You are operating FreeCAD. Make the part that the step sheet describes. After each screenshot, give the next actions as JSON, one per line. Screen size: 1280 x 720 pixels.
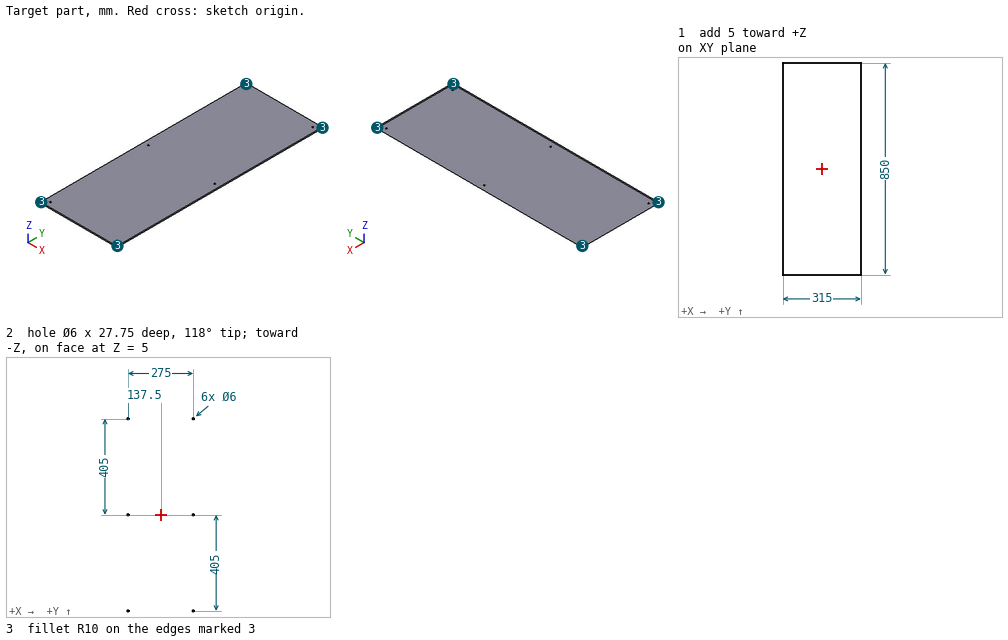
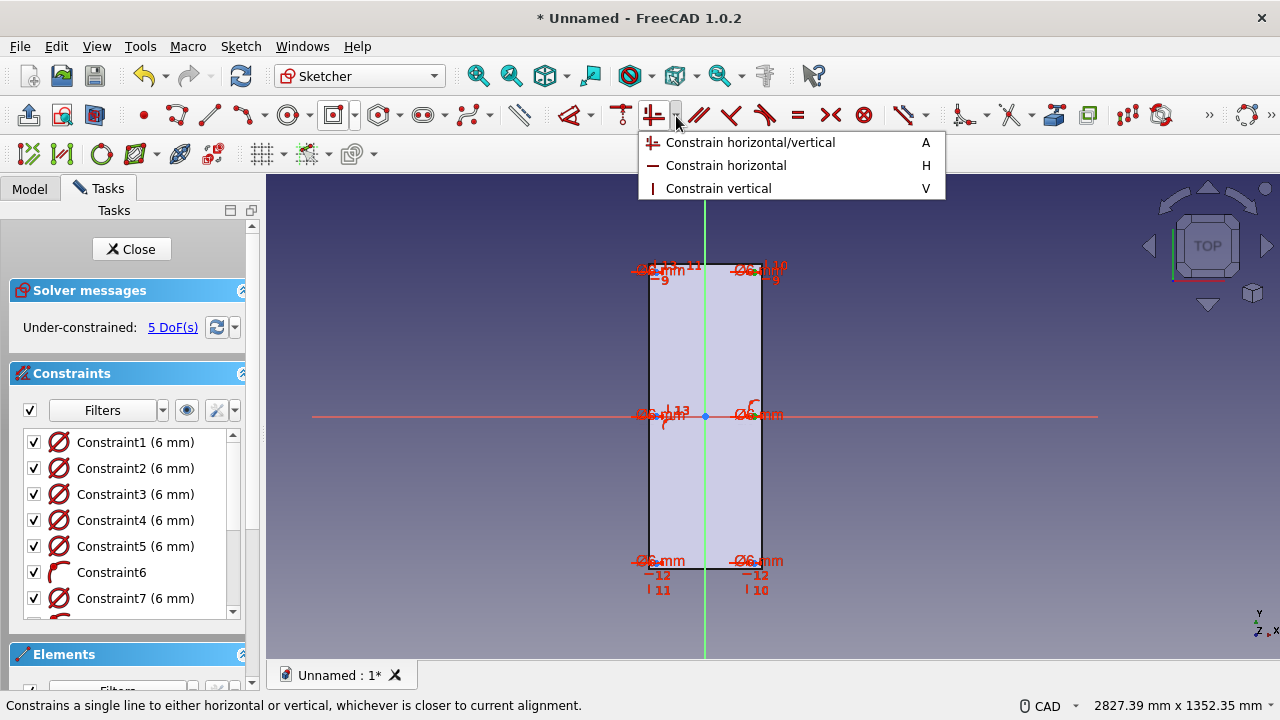
{"action": "left_click", "coordinate": [792, 188]}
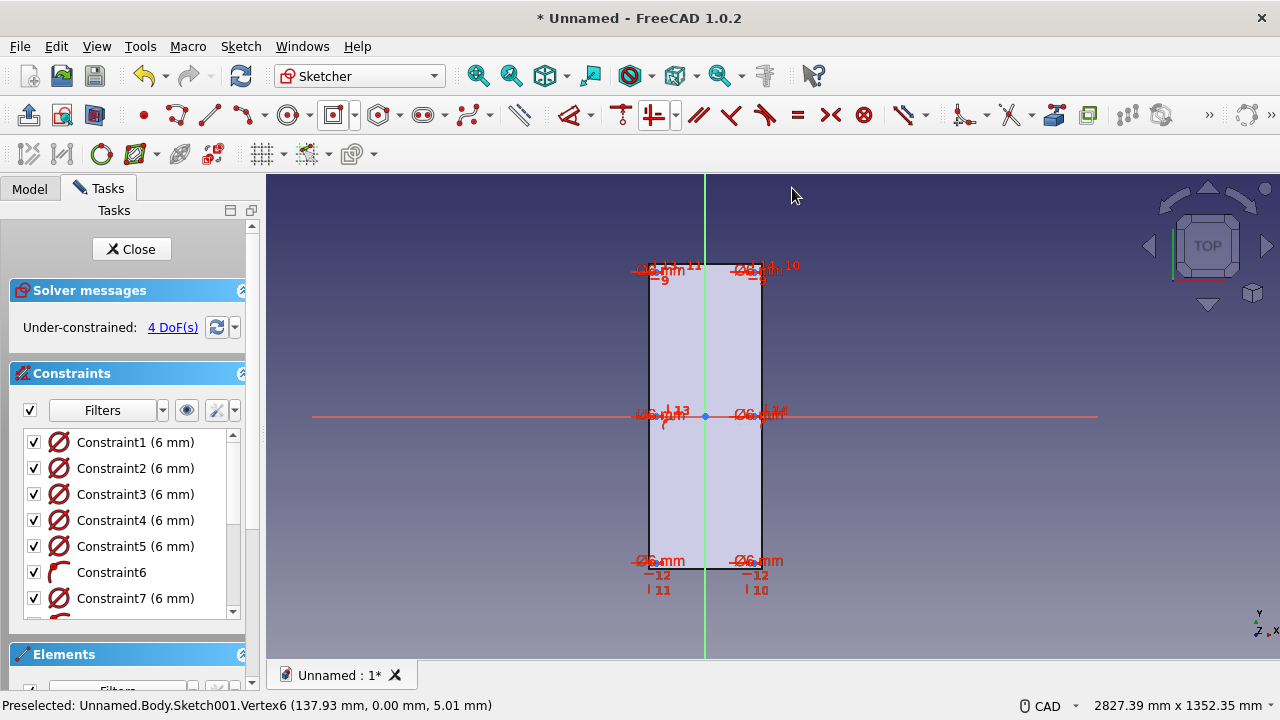
{"action": "key", "text": "d"}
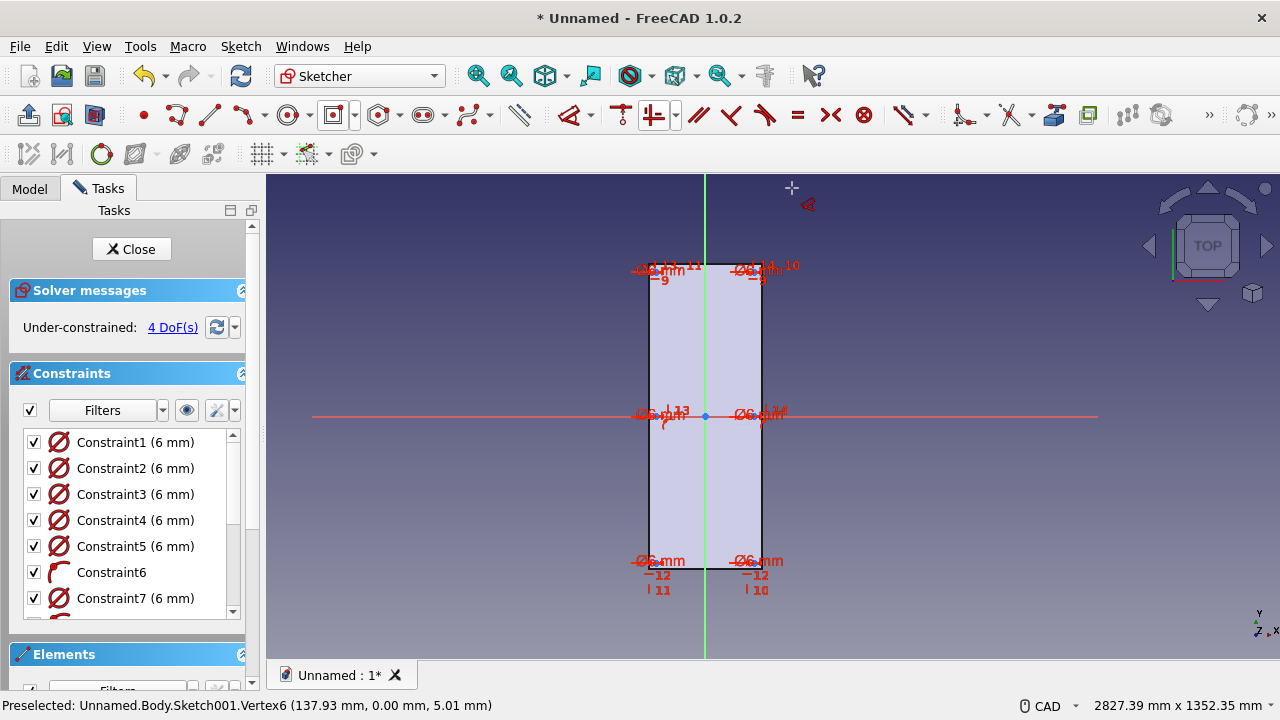
{"action": "left_click", "coordinate": [656, 272]}
{"action": "left_click", "coordinate": [622, 345]}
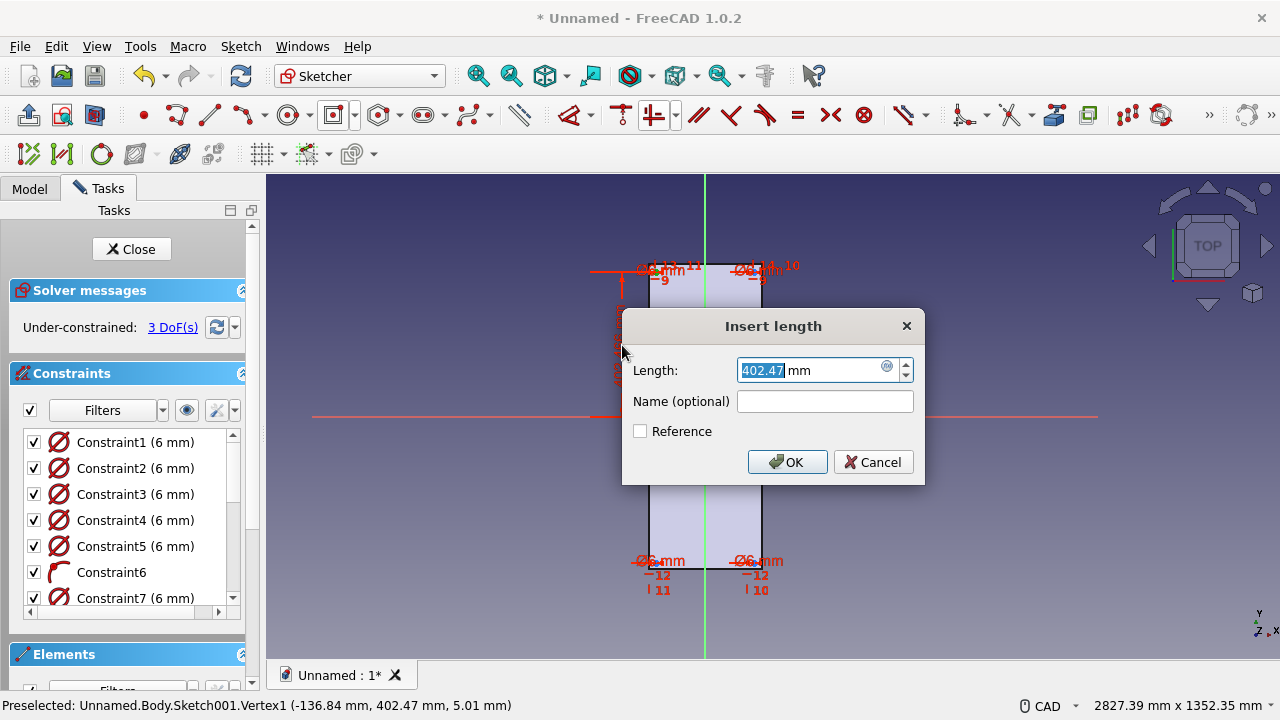
{"action": "type", "text": "405"}
{"action": "key", "text": "Return"}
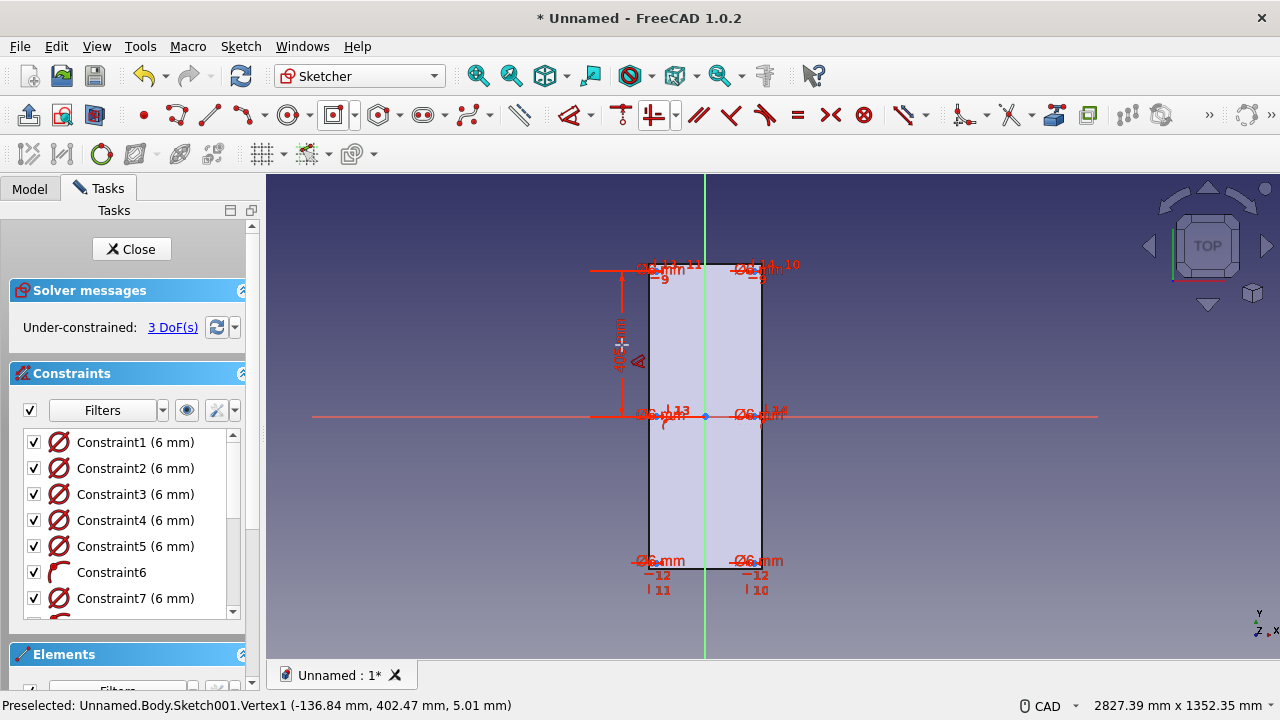
{"action": "left_click", "coordinate": [754, 563]}
{"action": "left_click", "coordinate": [788, 490]}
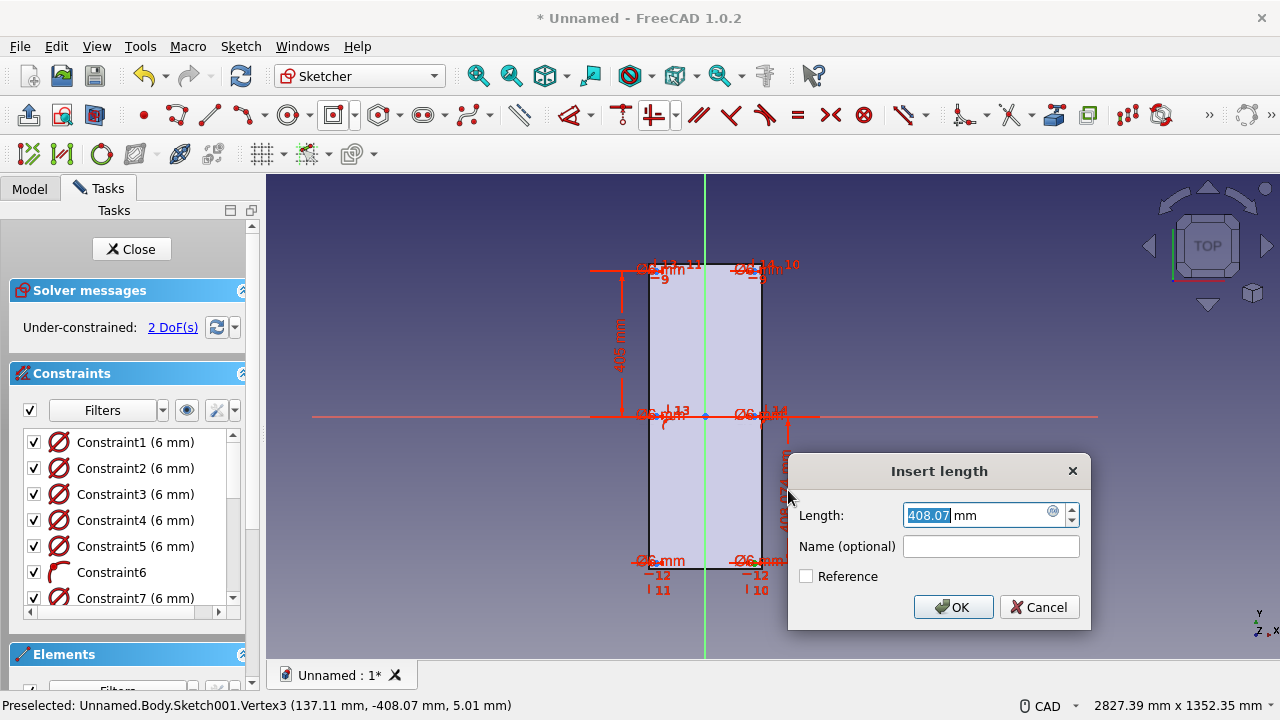
{"action": "type", "text": "405"}
{"action": "key", "text": "Return"}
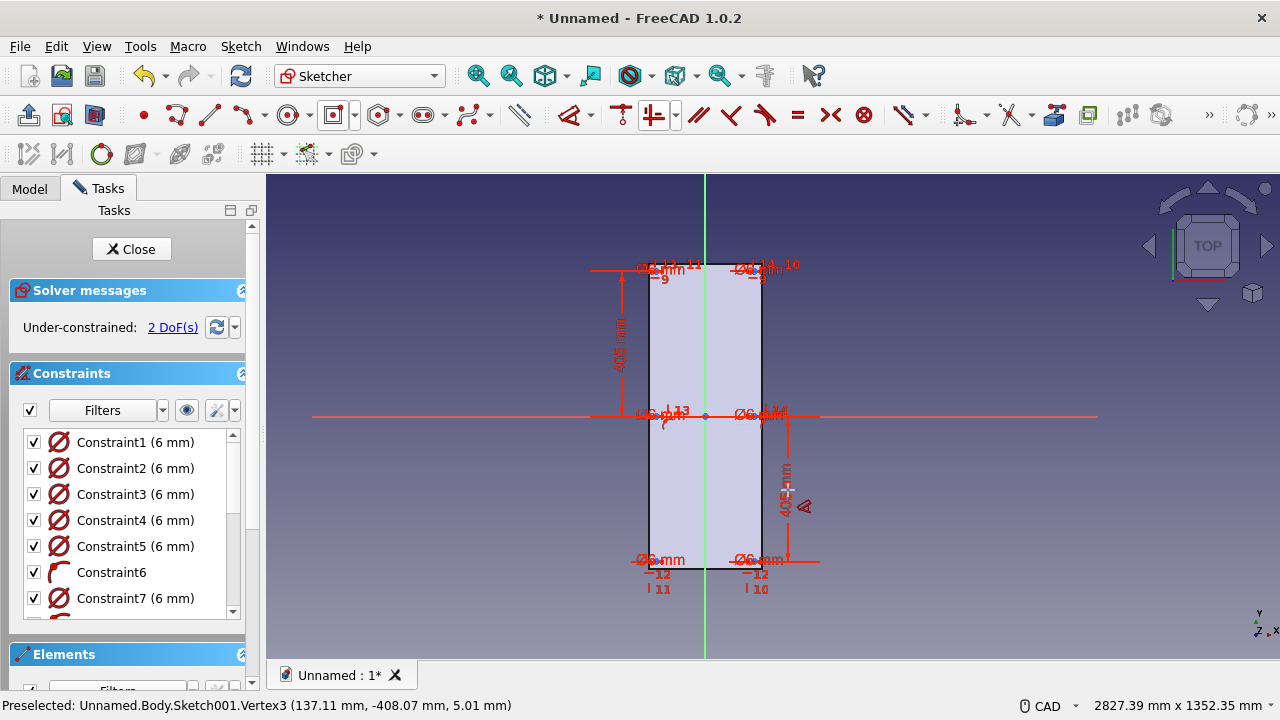
{"action": "left_click", "coordinate": [656, 271]}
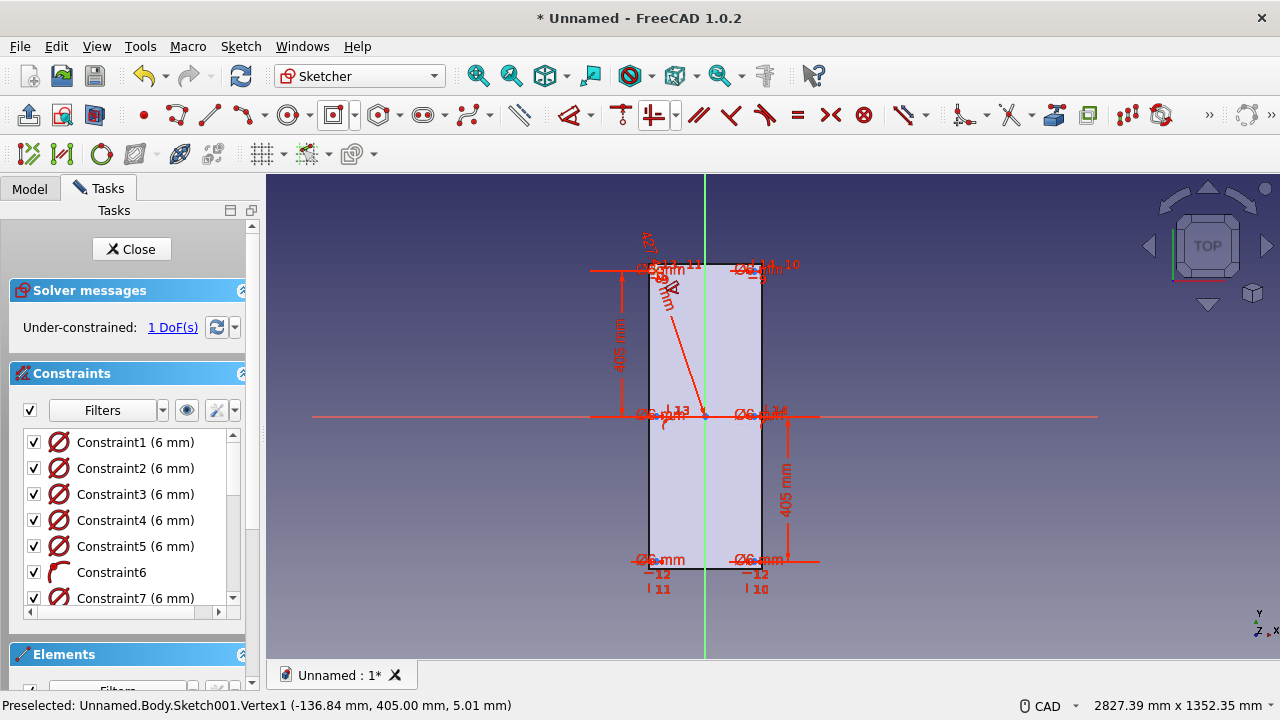
{"action": "left_click", "coordinate": [754, 271]}
{"action": "left_click", "coordinate": [683, 237]}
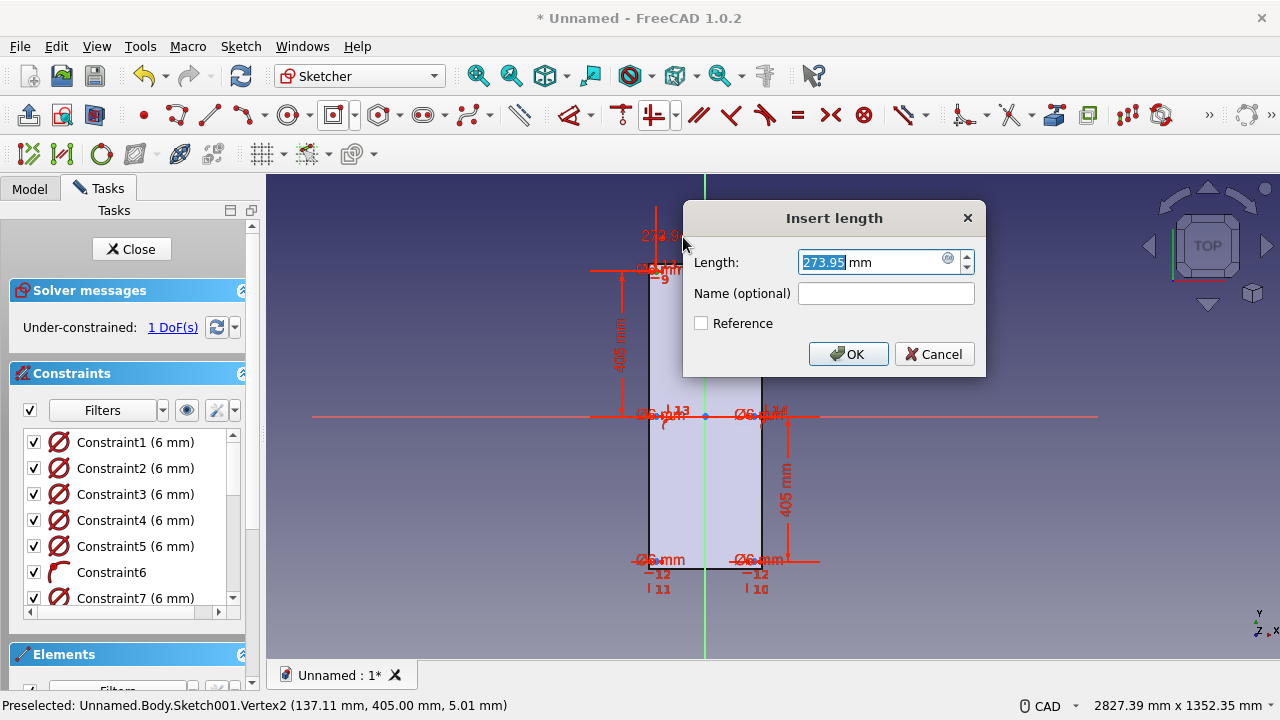
{"action": "type", "text": "275"}
{"action": "key", "text": "Return"}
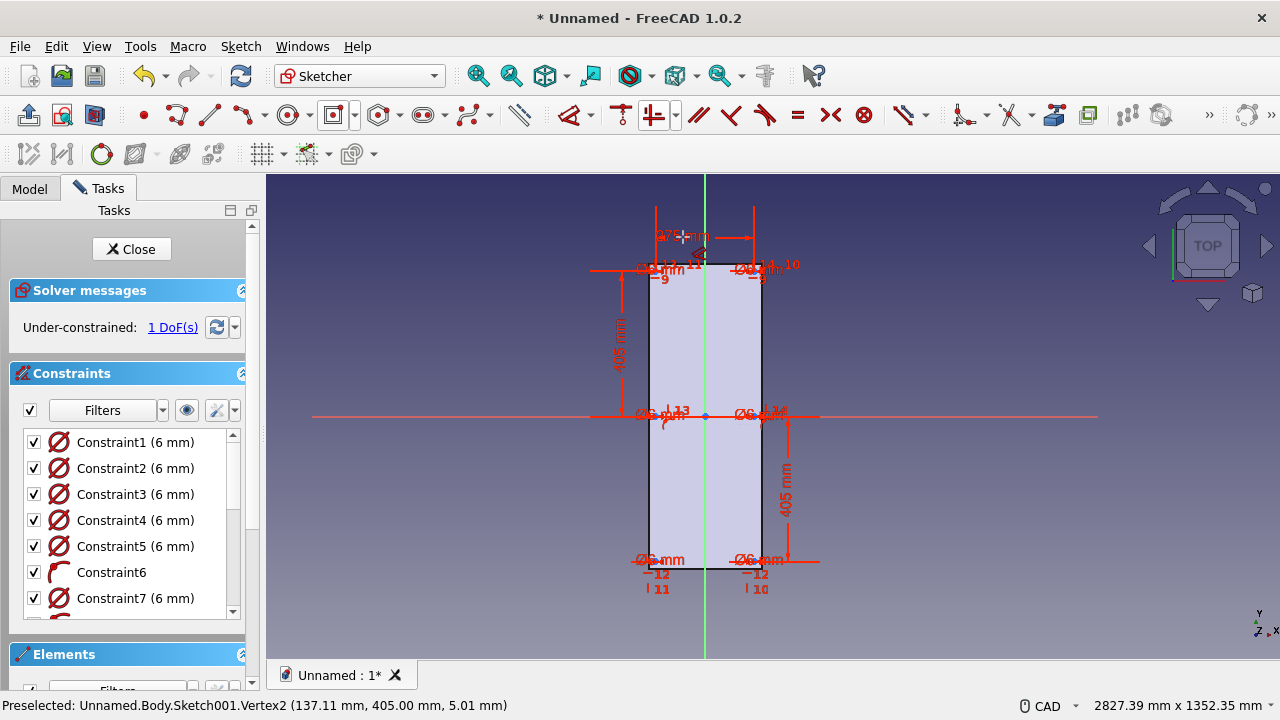
{"action": "left_click", "coordinate": [656, 271]}
{"action": "left_click", "coordinate": [680, 451]}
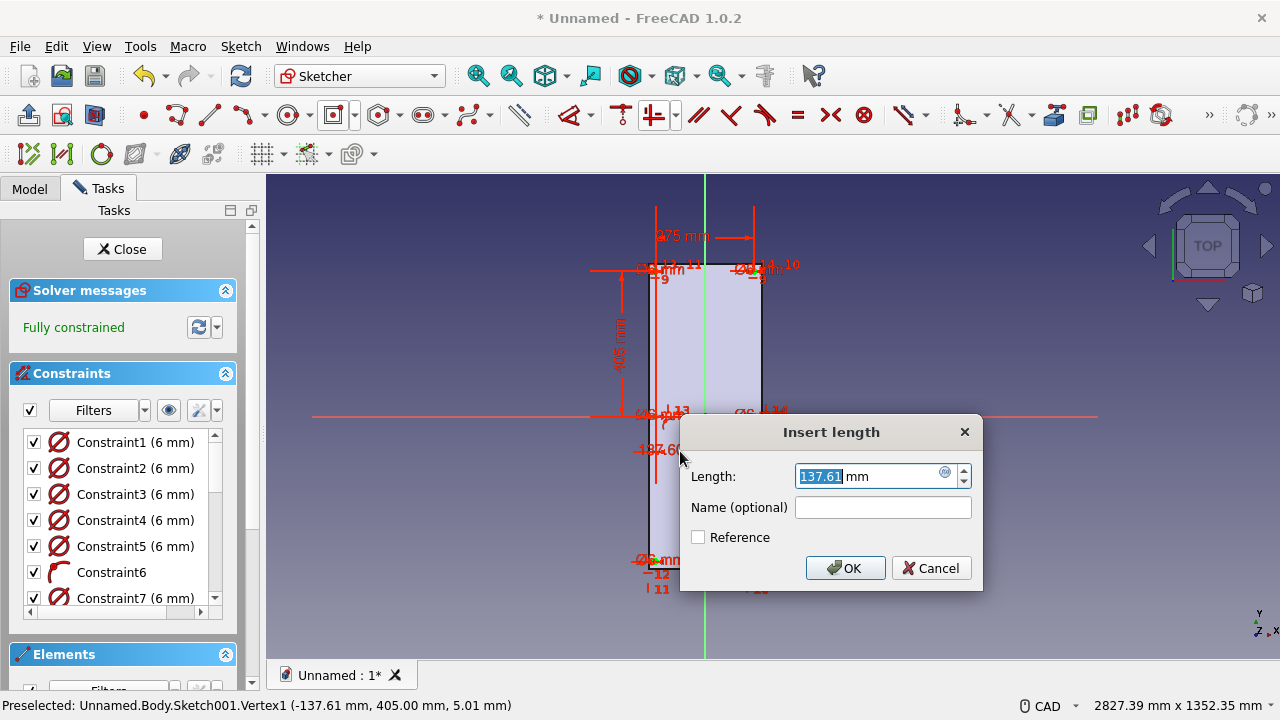
{"action": "type", "text": "137.5"}
{"action": "key", "text": "Return"}
{"action": "key", "text": "Escape"}